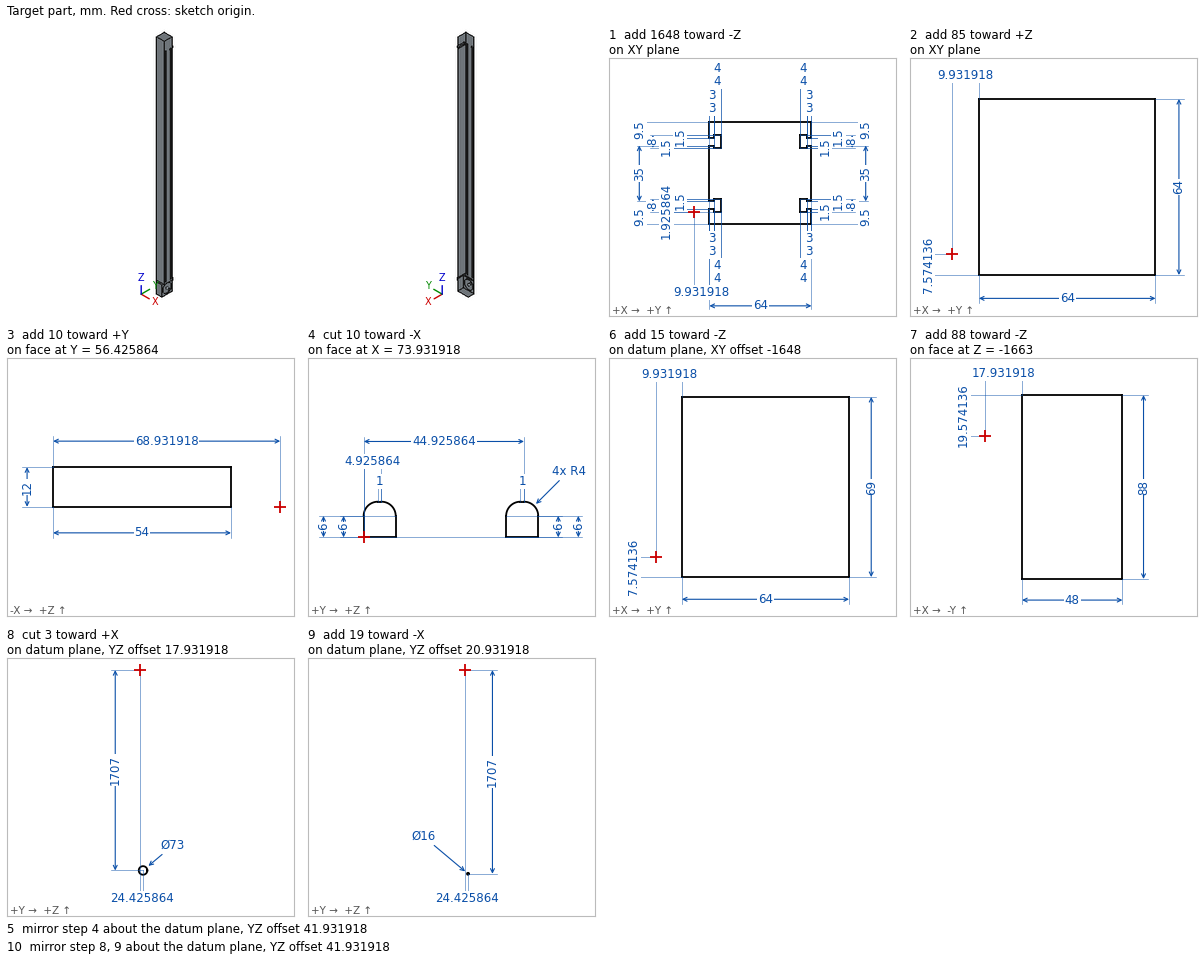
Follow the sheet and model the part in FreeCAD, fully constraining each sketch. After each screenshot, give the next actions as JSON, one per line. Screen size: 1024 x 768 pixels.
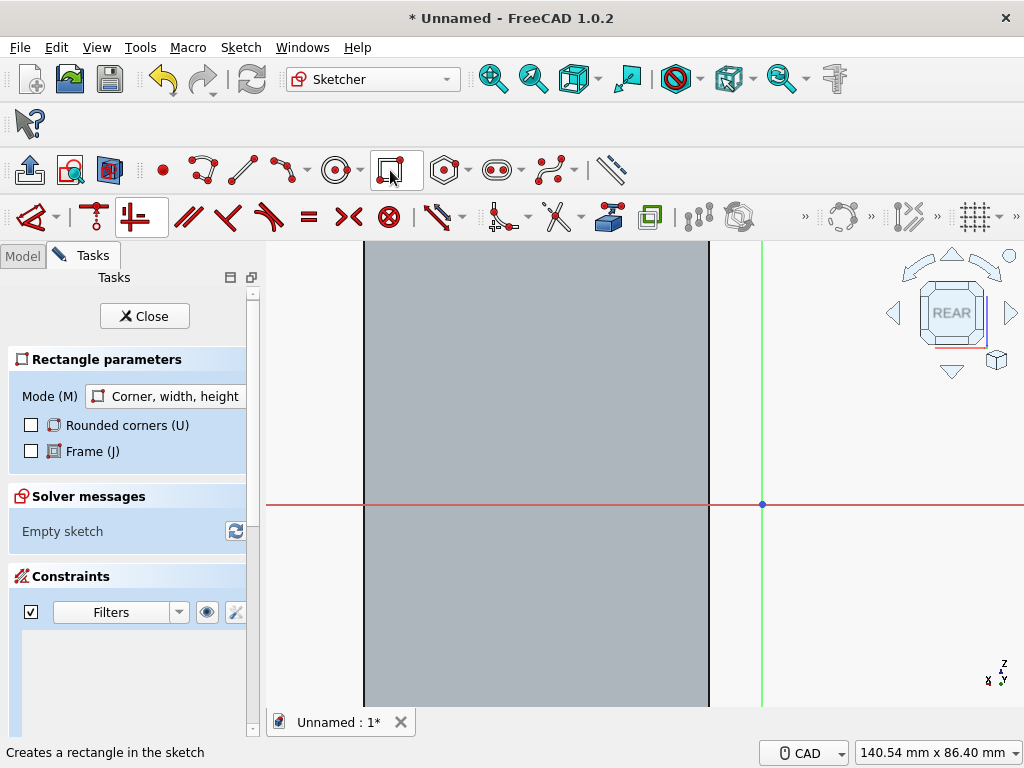
{"action": "left_click", "coordinate": [391, 440]}
{"action": "left_click", "coordinate": [682, 505]}
{"action": "key", "text": "Escape"}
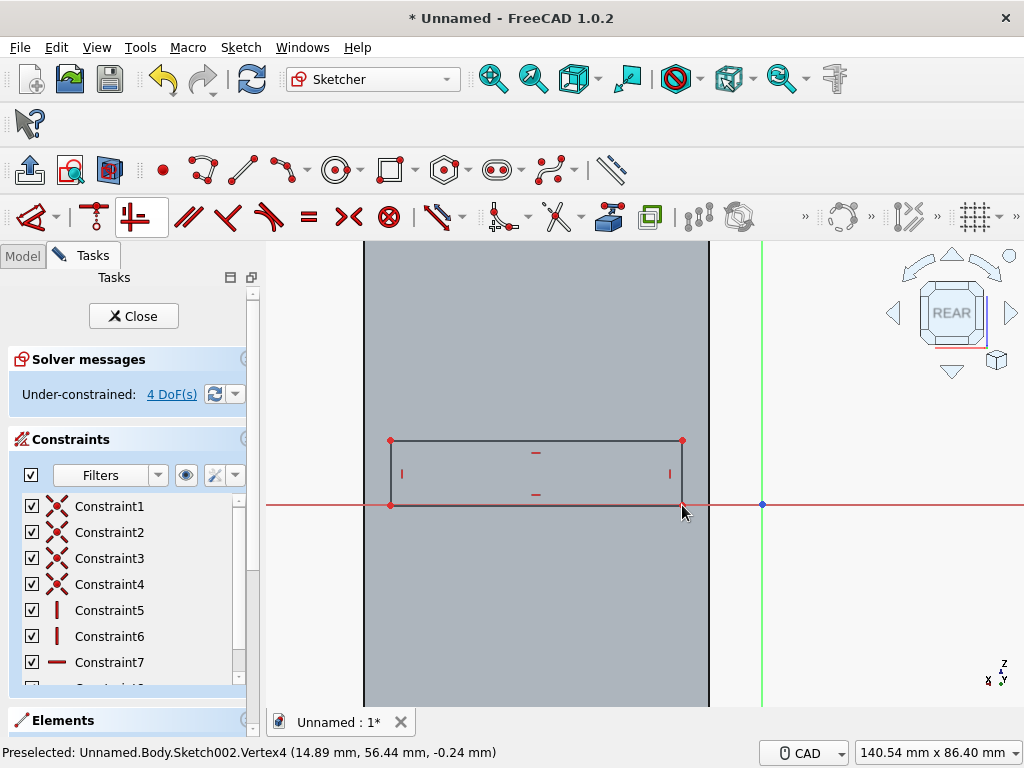
{"action": "left_click", "coordinate": [391, 506]}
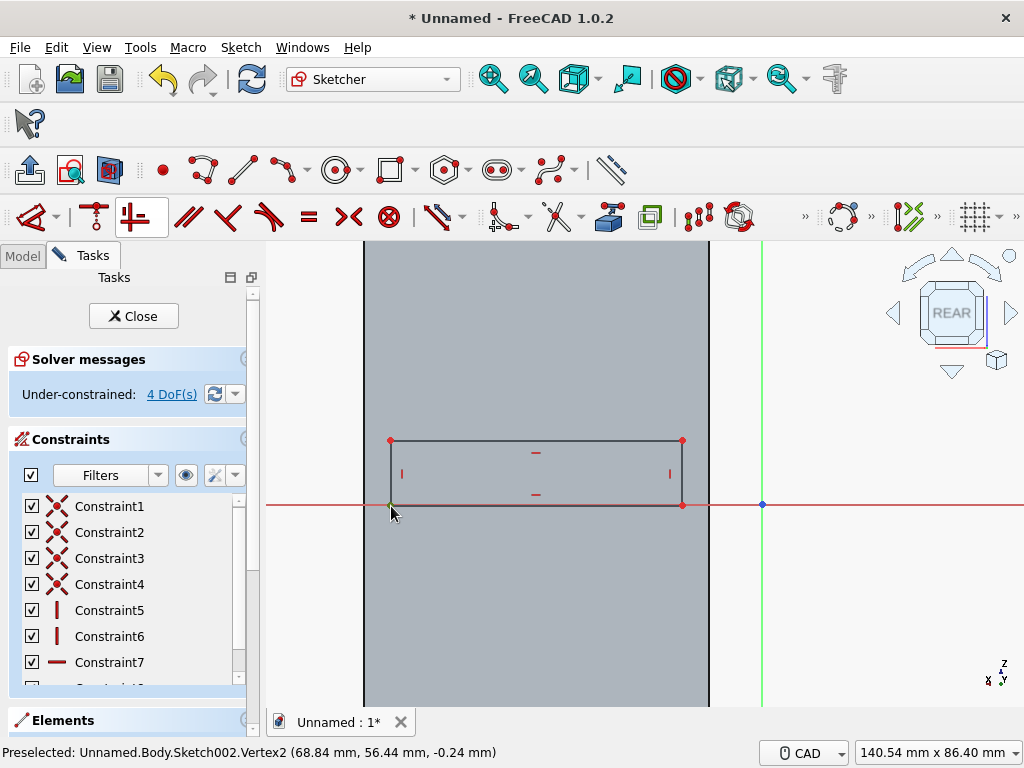
{"action": "left_click", "coordinate": [334, 505]}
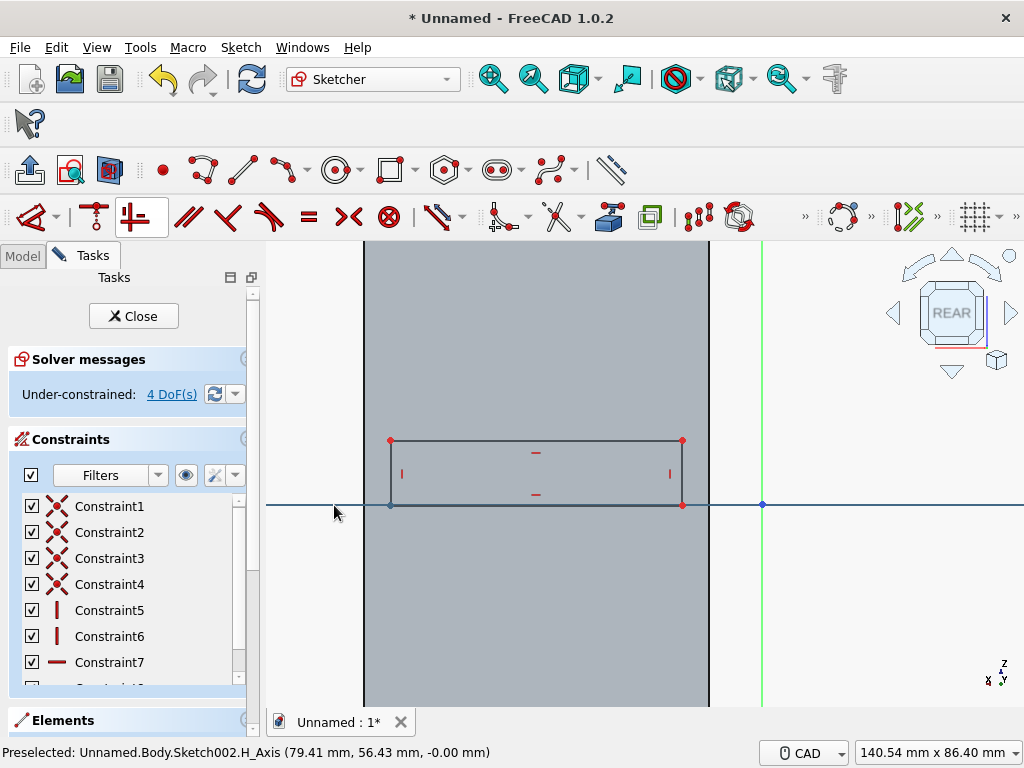
{"action": "left_click", "coordinate": [94, 218]}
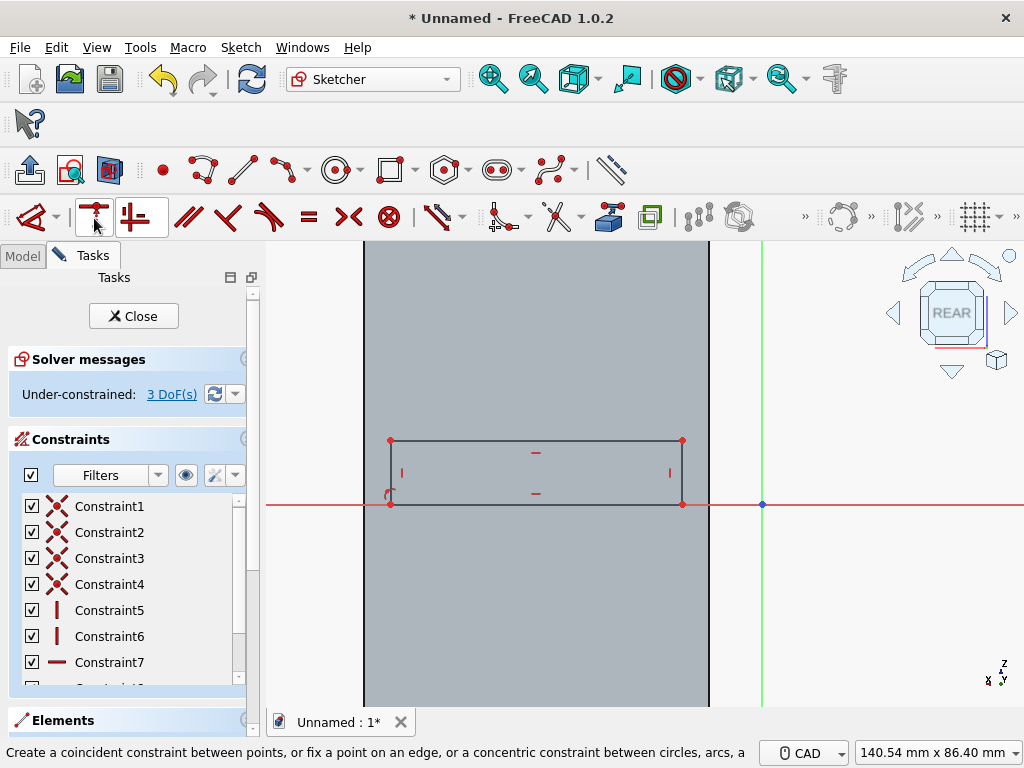
{"action": "left_click", "coordinate": [32, 218]}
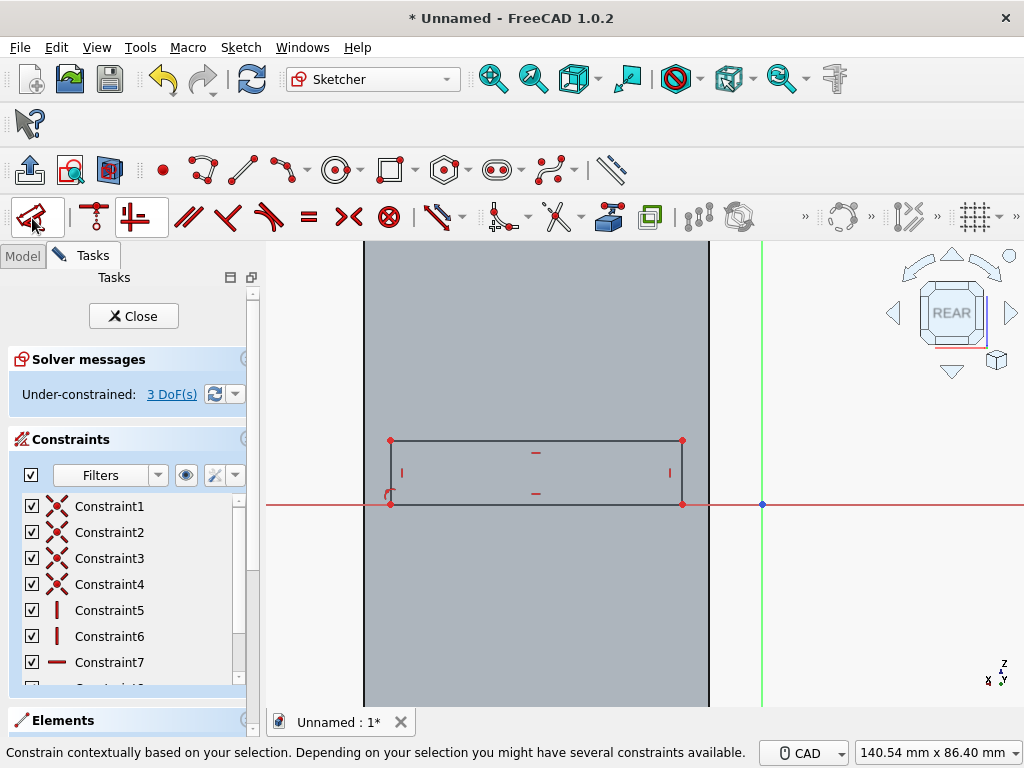
{"action": "left_click", "coordinate": [391, 460]}
{"action": "left_click", "coordinate": [357, 473]}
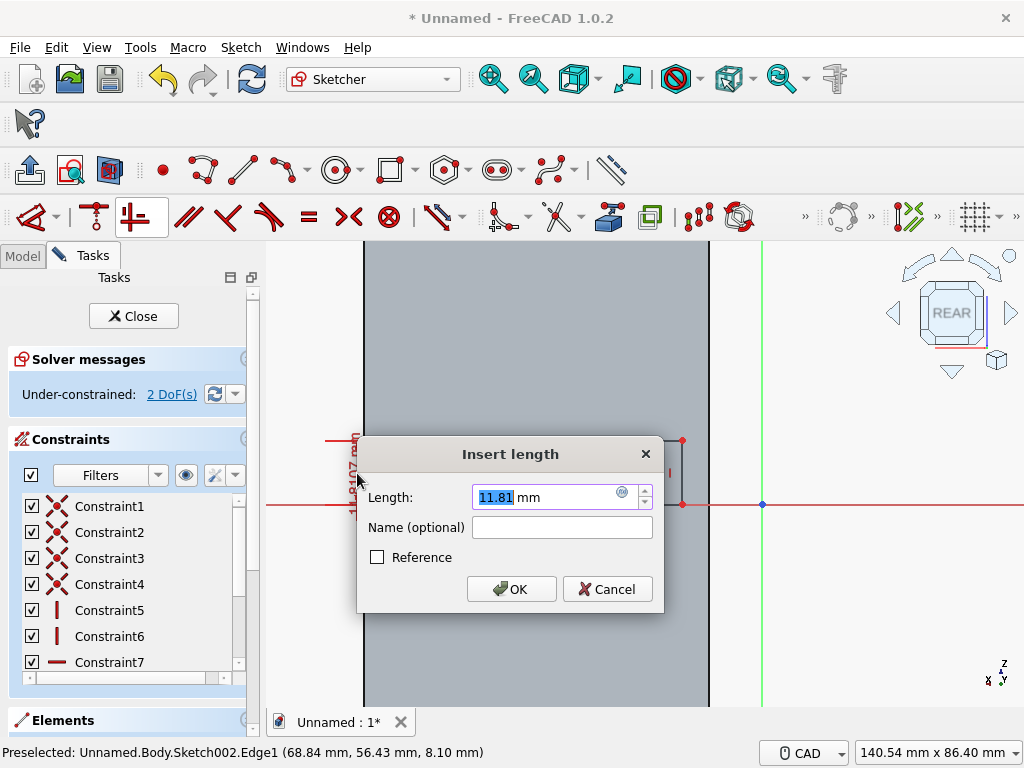
{"action": "type", "text": "12"}
{"action": "key", "text": "Return"}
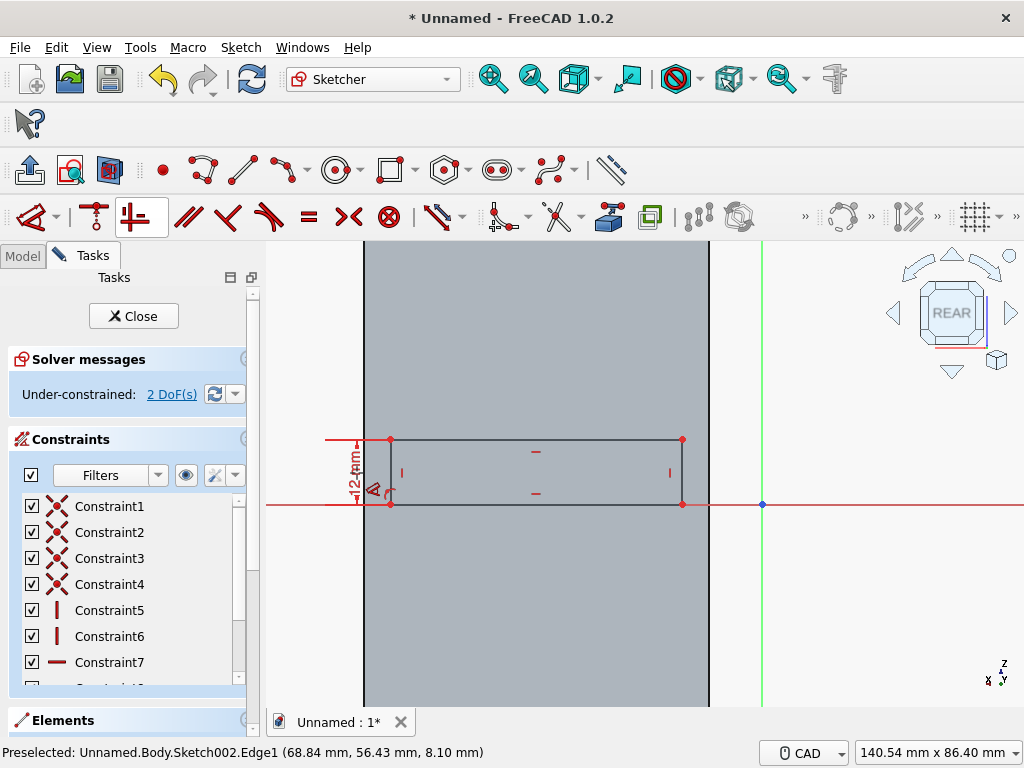
{"action": "left_click", "coordinate": [478, 505]}
{"action": "left_click", "coordinate": [537, 539]}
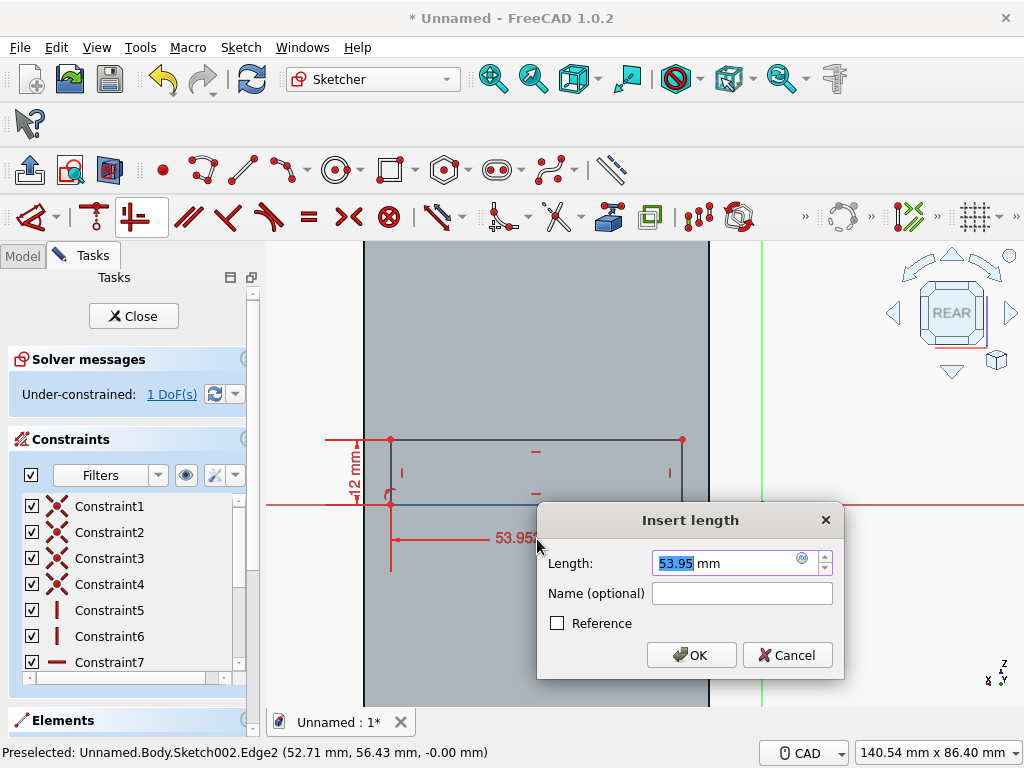
{"action": "type", "text": "54"}
{"action": "key", "text": "Return"}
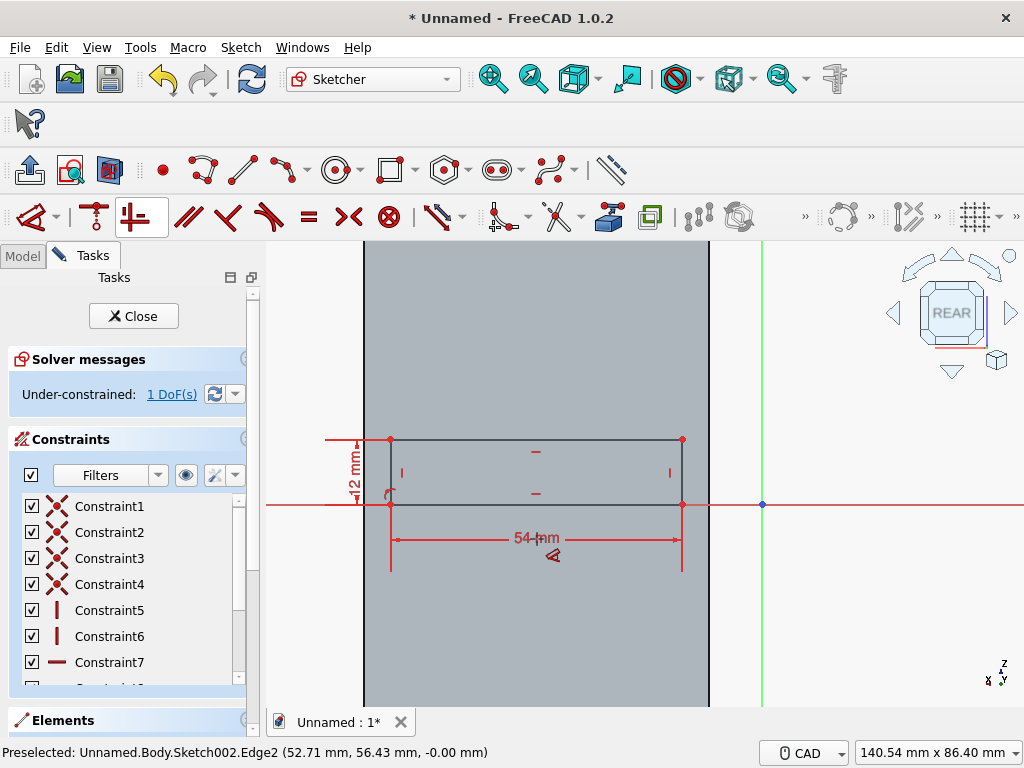
{"action": "left_click", "coordinate": [391, 440]}
{"action": "left_click", "coordinate": [662, 539]}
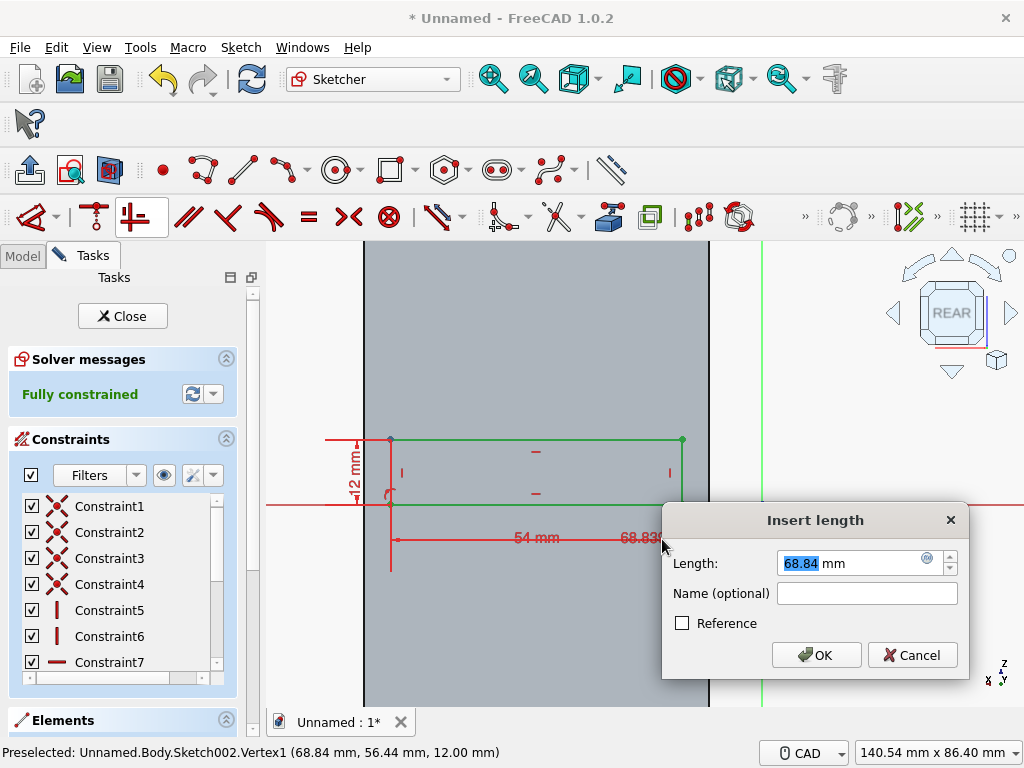
{"action": "type", "text": "68.931918"}
{"action": "key", "text": "Return"}
{"action": "key", "text": "Escape"}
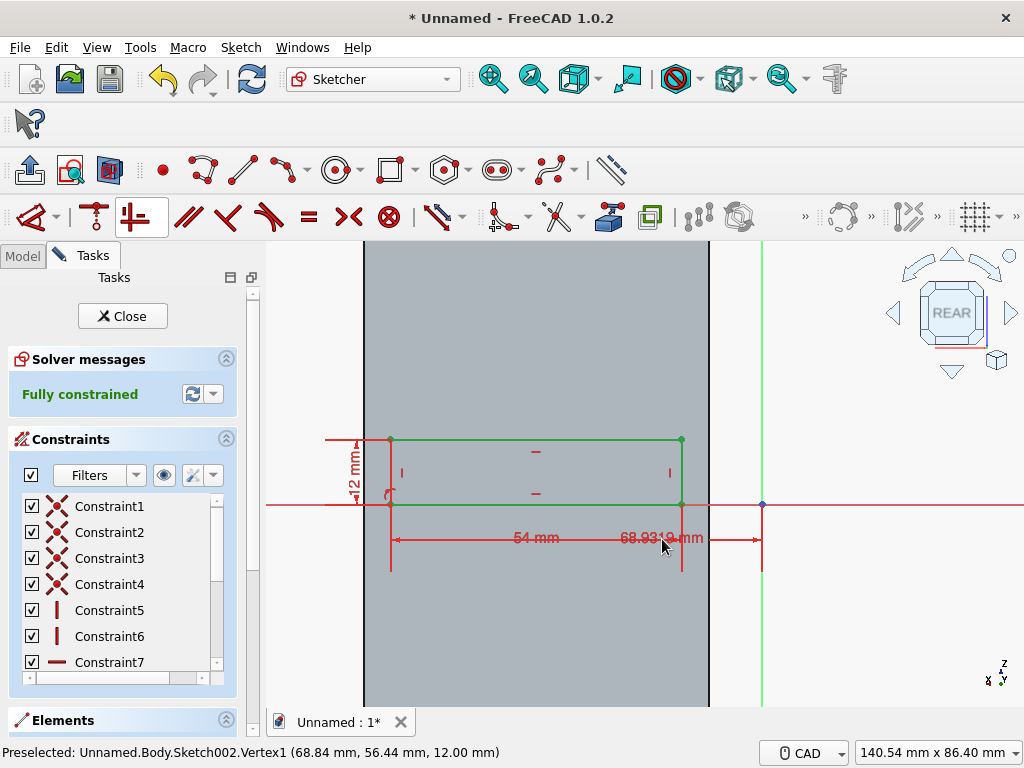
{"action": "left_click", "coordinate": [123, 316]}